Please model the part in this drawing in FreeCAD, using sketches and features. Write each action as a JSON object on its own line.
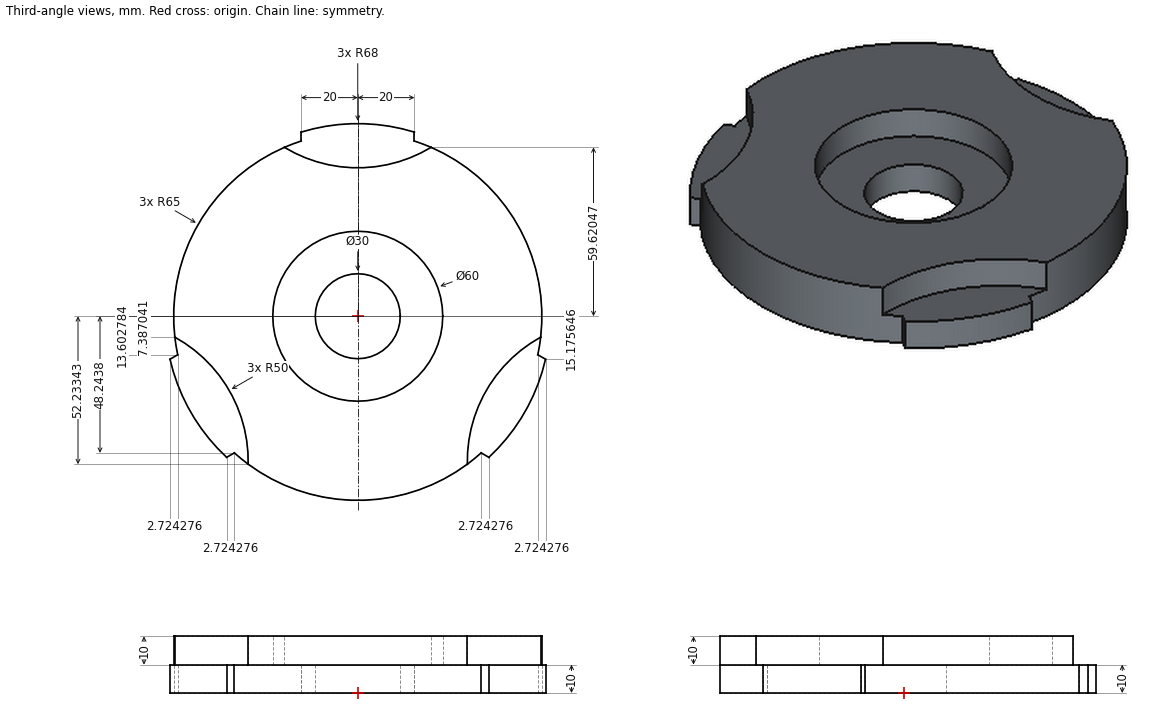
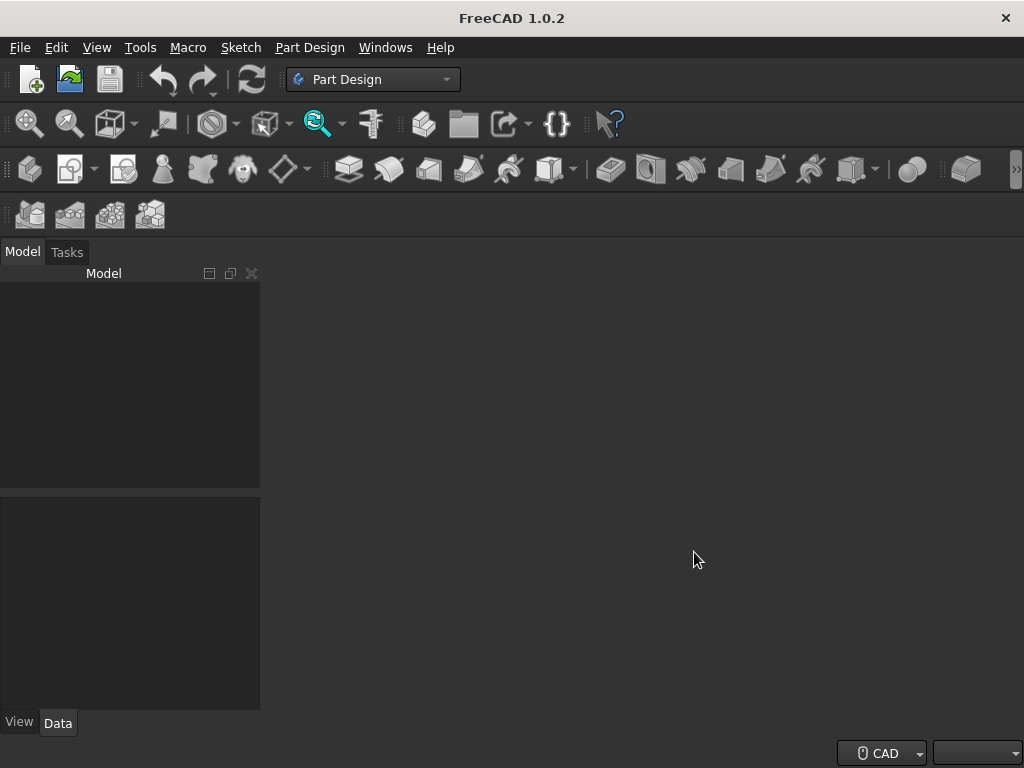
{"action": "left_click", "coordinate": [30, 80]}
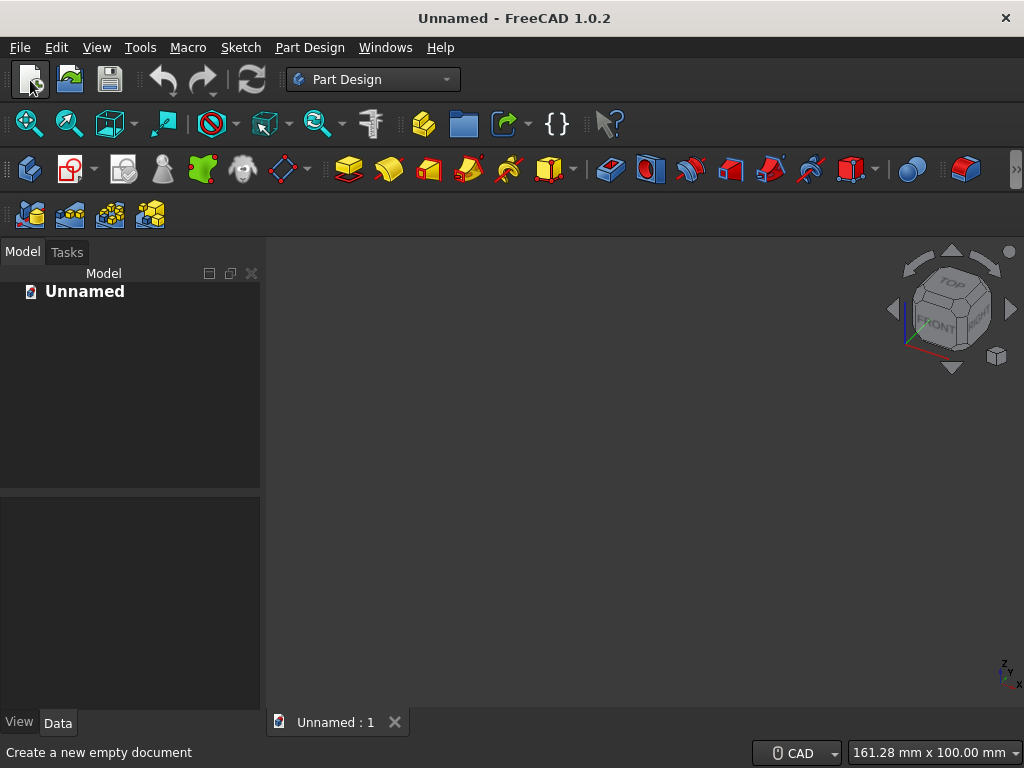
{"action": "left_click", "coordinate": [70, 170]}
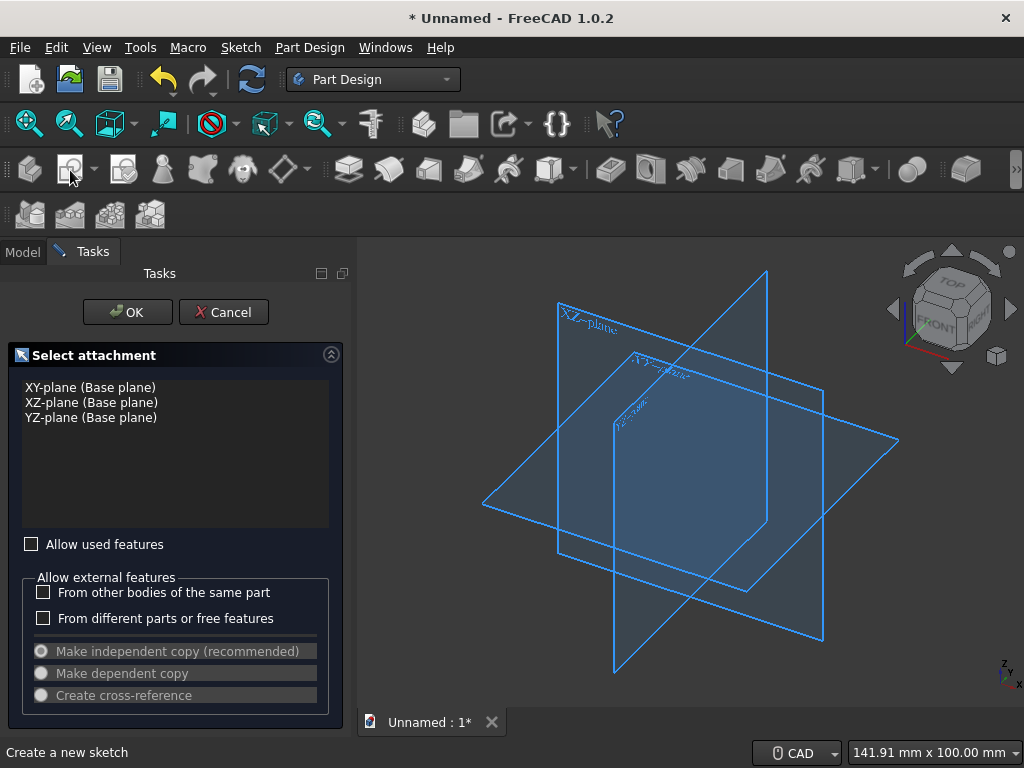
{"action": "left_click", "coordinate": [82, 388]}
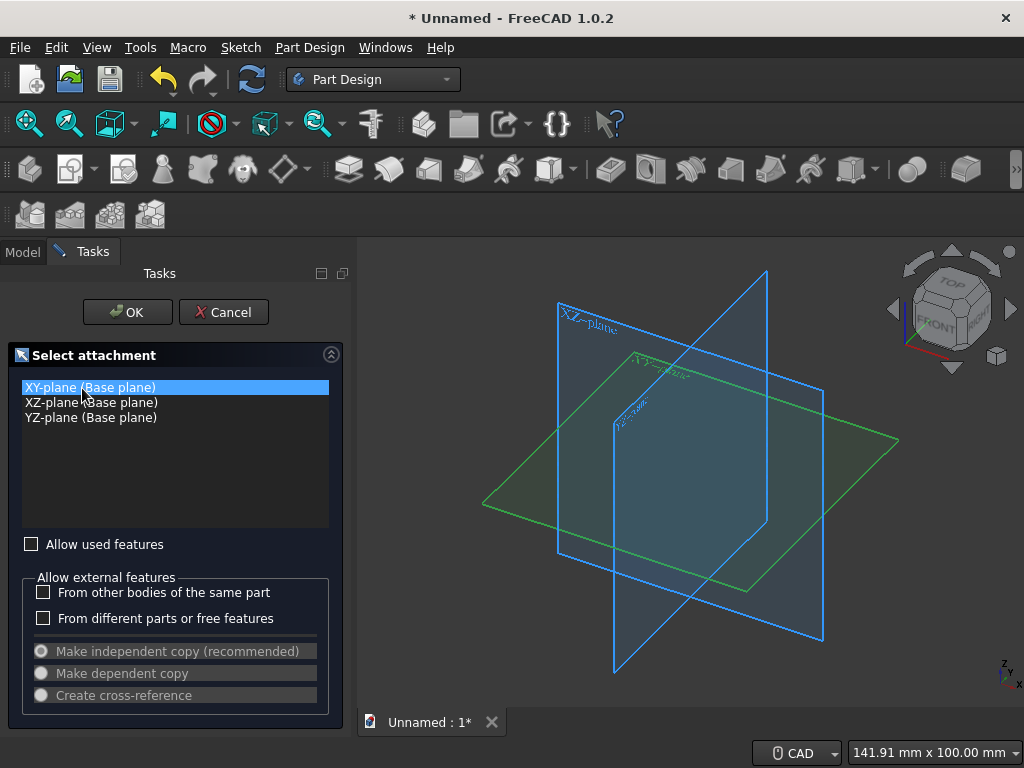
{"action": "left_click", "coordinate": [128, 312]}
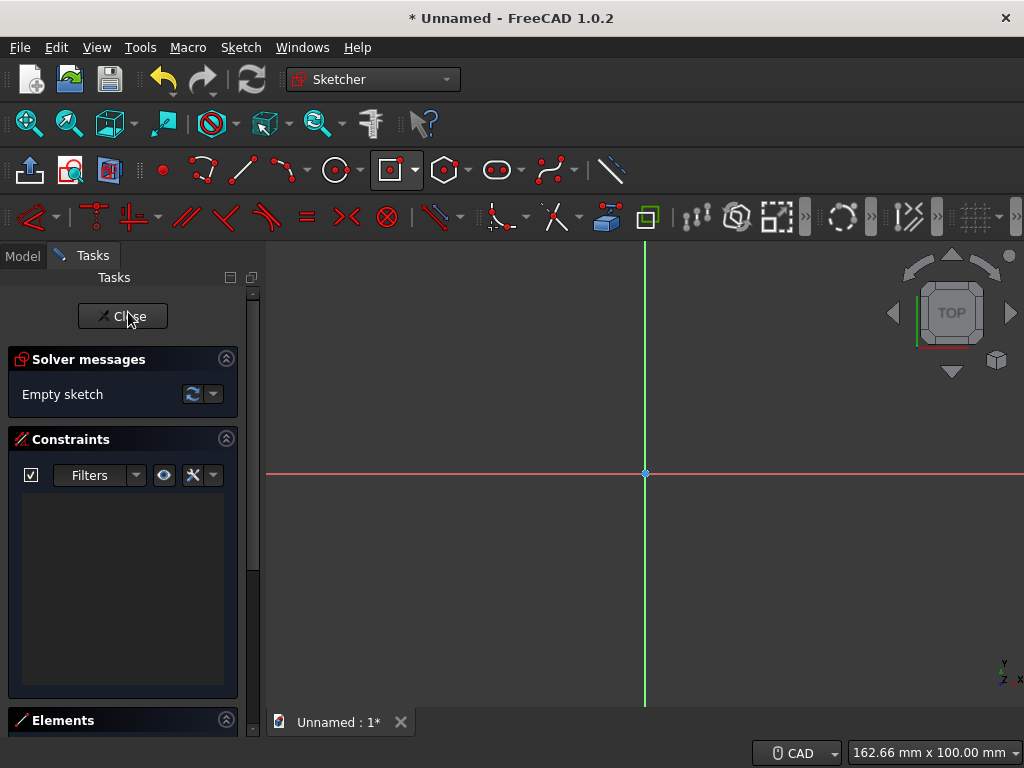
{"action": "scroll", "coordinate": [521, 480], "scroll_direction": "down", "scroll_amount": 4}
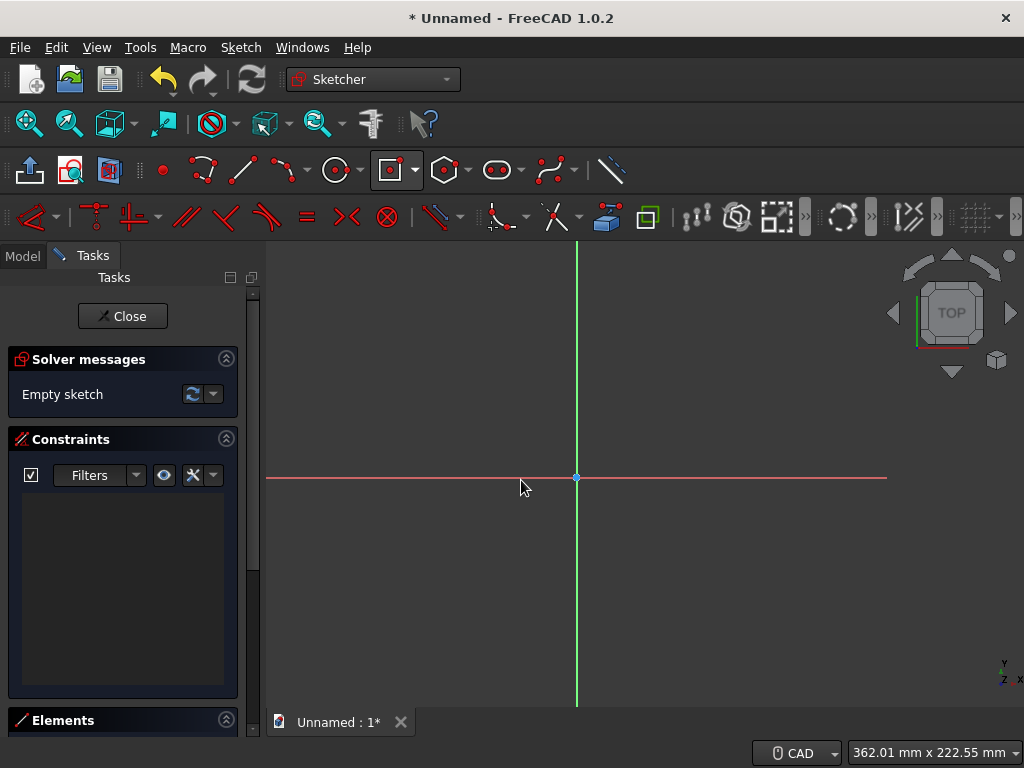
{"action": "left_click", "coordinate": [244, 170]}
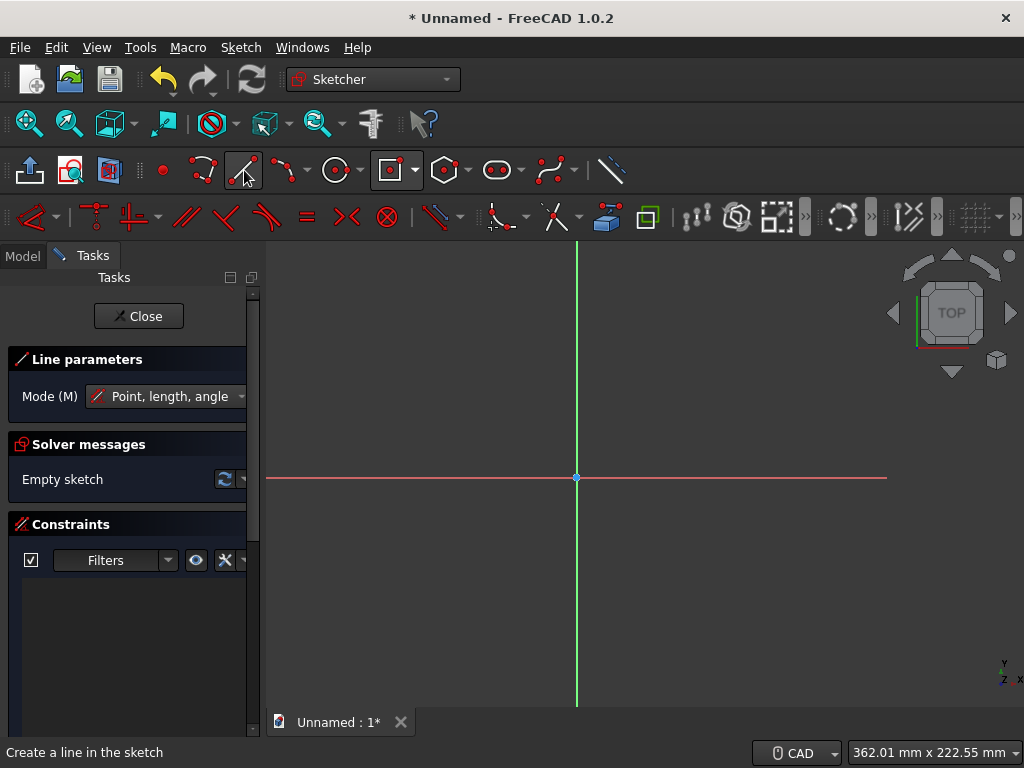
{"action": "left_click", "coordinate": [619, 348]}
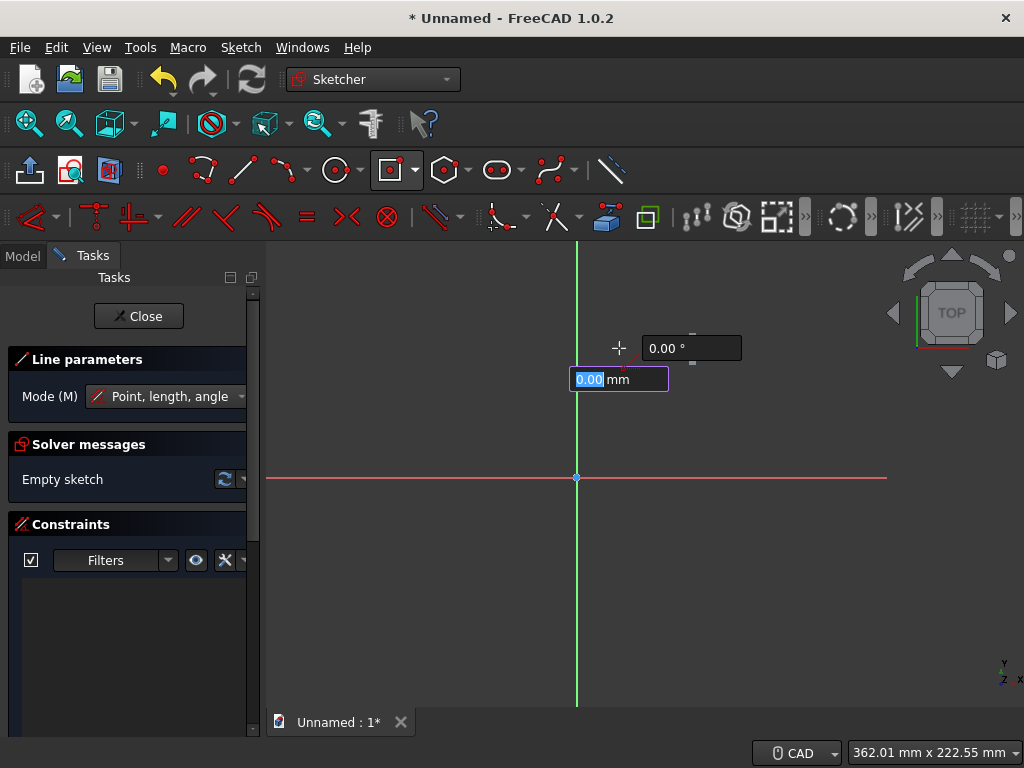
{"action": "scroll", "coordinate": [619, 342], "scroll_direction": "up", "scroll_amount": 5}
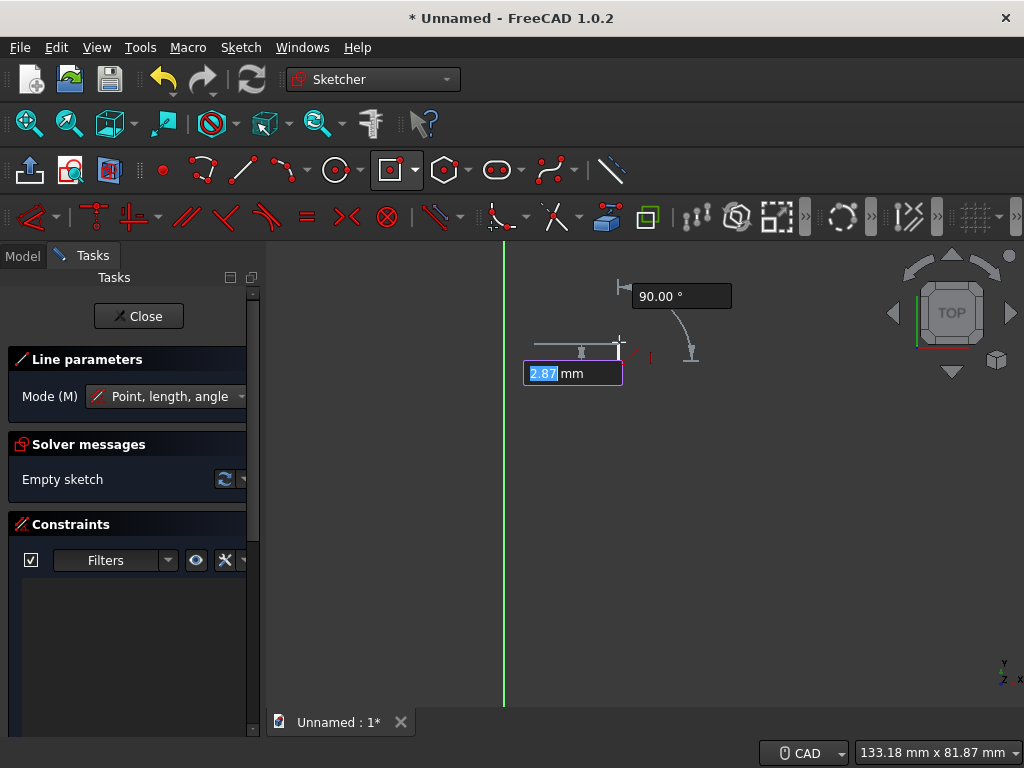
{"action": "left_click", "coordinate": [618, 340]}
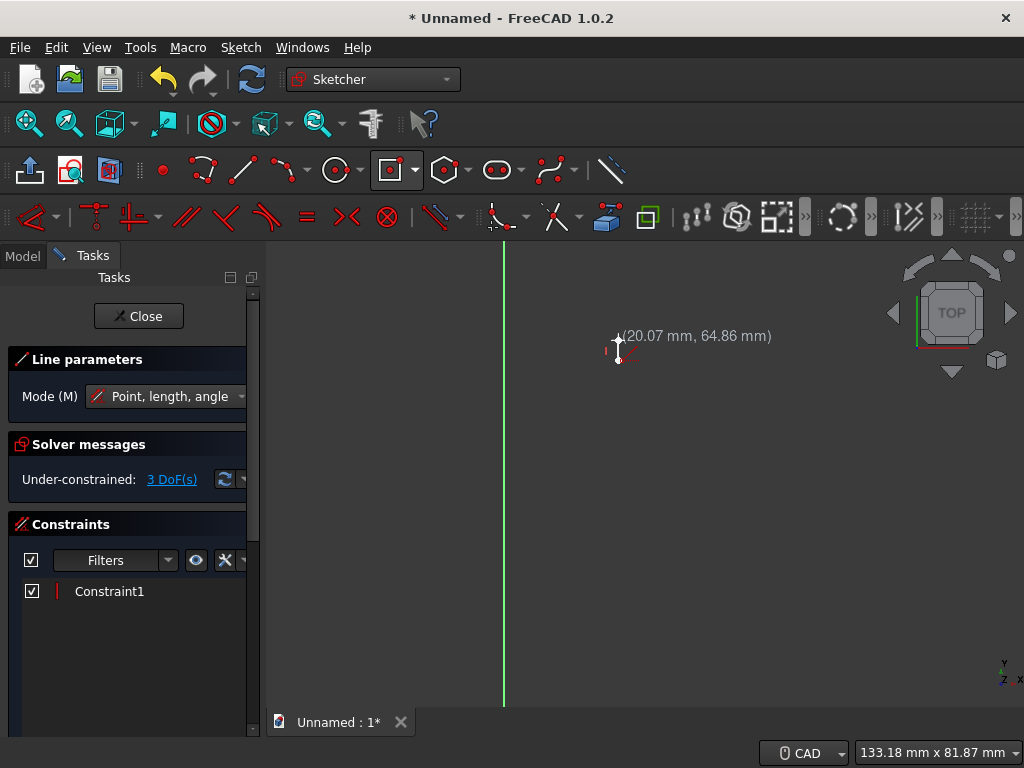
{"action": "left_click", "coordinate": [390, 340]}
{"action": "left_click", "coordinate": [390, 358]}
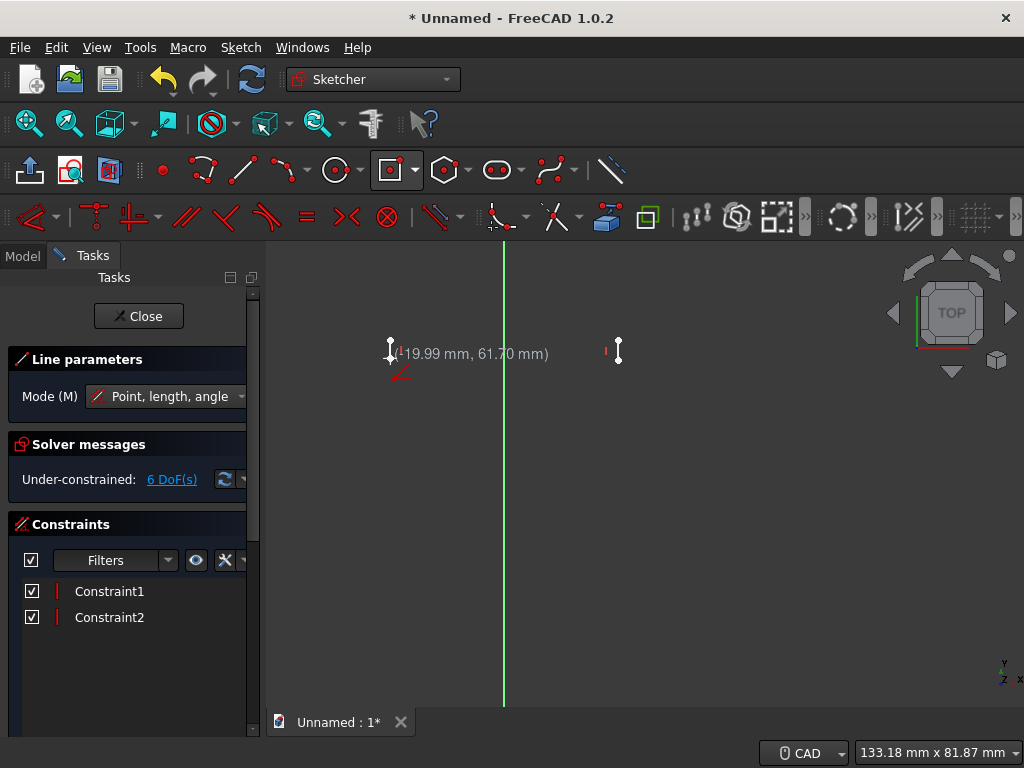
{"action": "scroll", "coordinate": [619, 342], "scroll_direction": "down", "scroll_amount": 5}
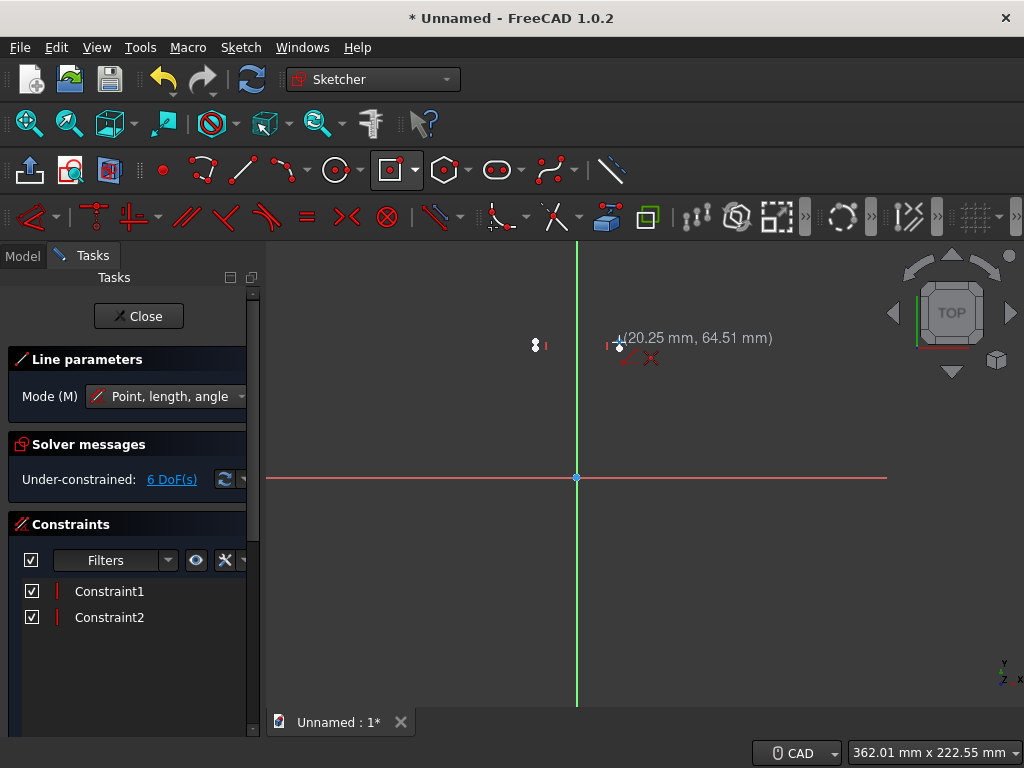
{"action": "left_click", "coordinate": [444, 506]}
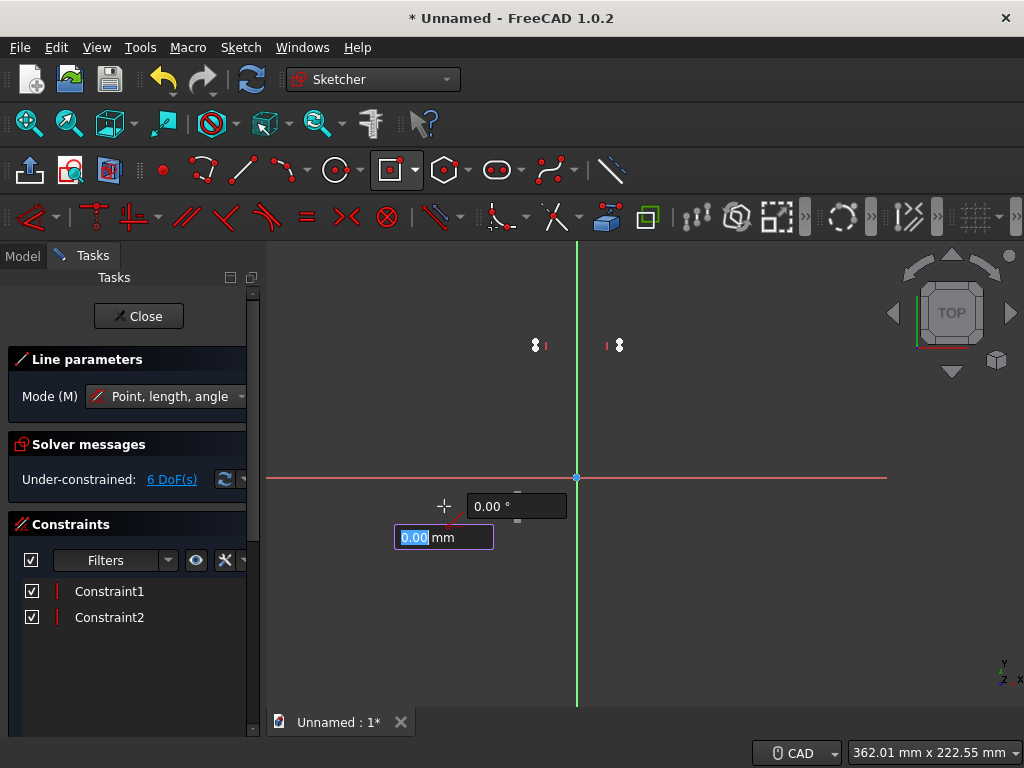
{"action": "scroll", "coordinate": [438, 509], "scroll_direction": "up", "scroll_amount": 5}